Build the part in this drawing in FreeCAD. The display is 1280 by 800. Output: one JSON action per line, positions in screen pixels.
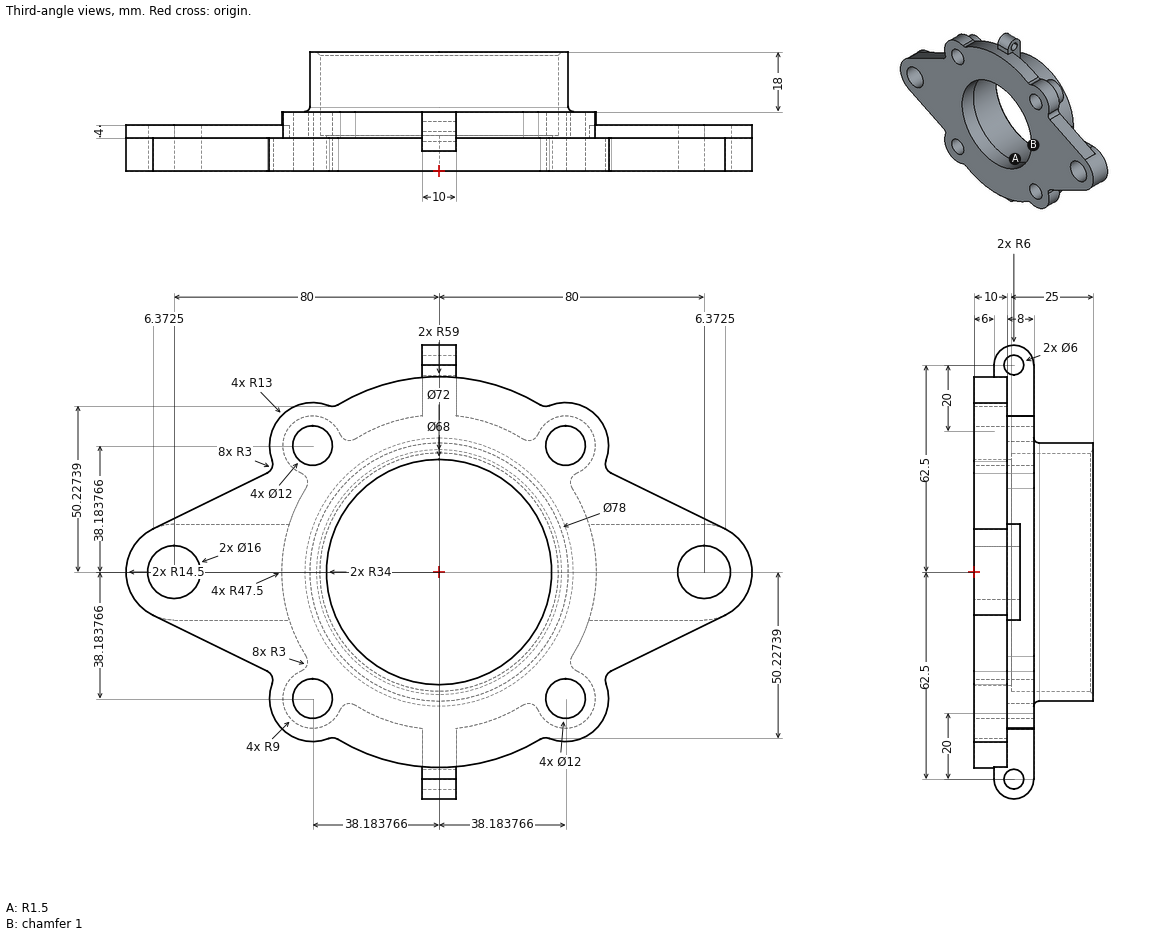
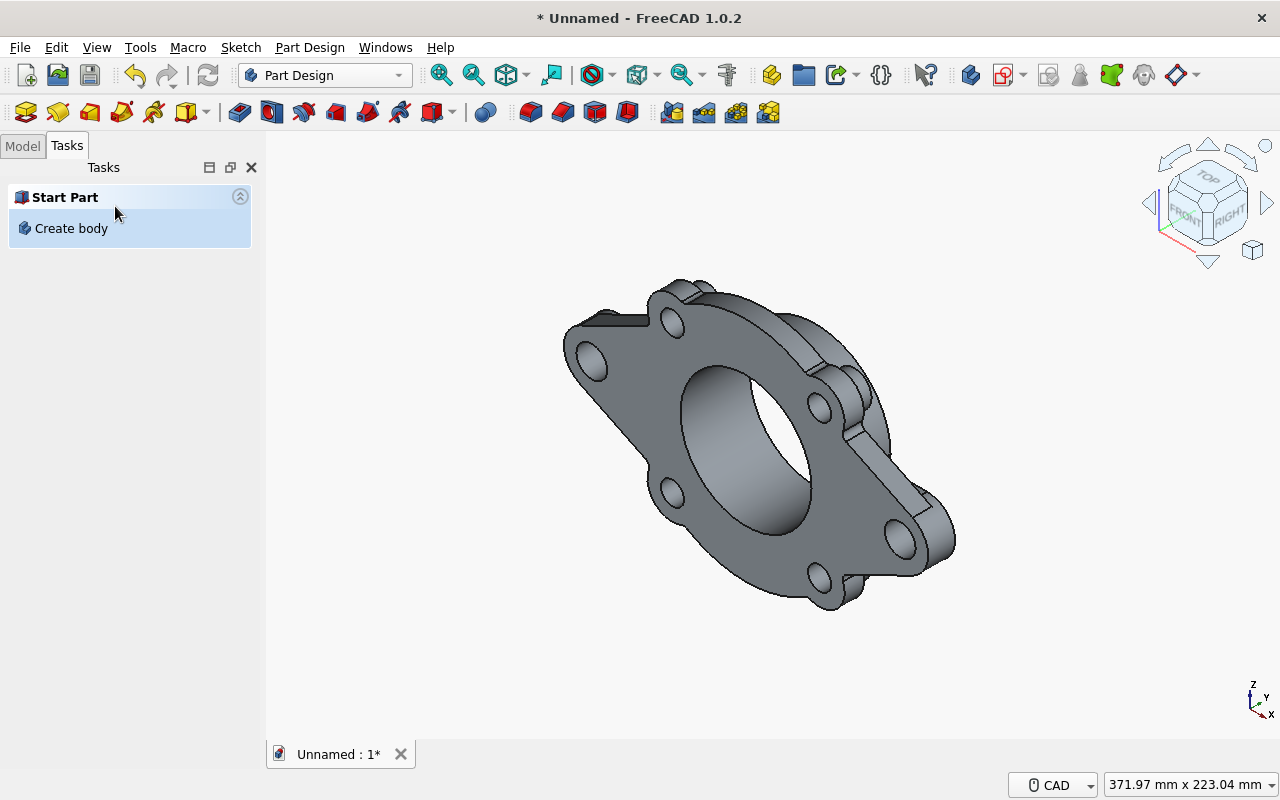
{"action": "key", "text": "2"}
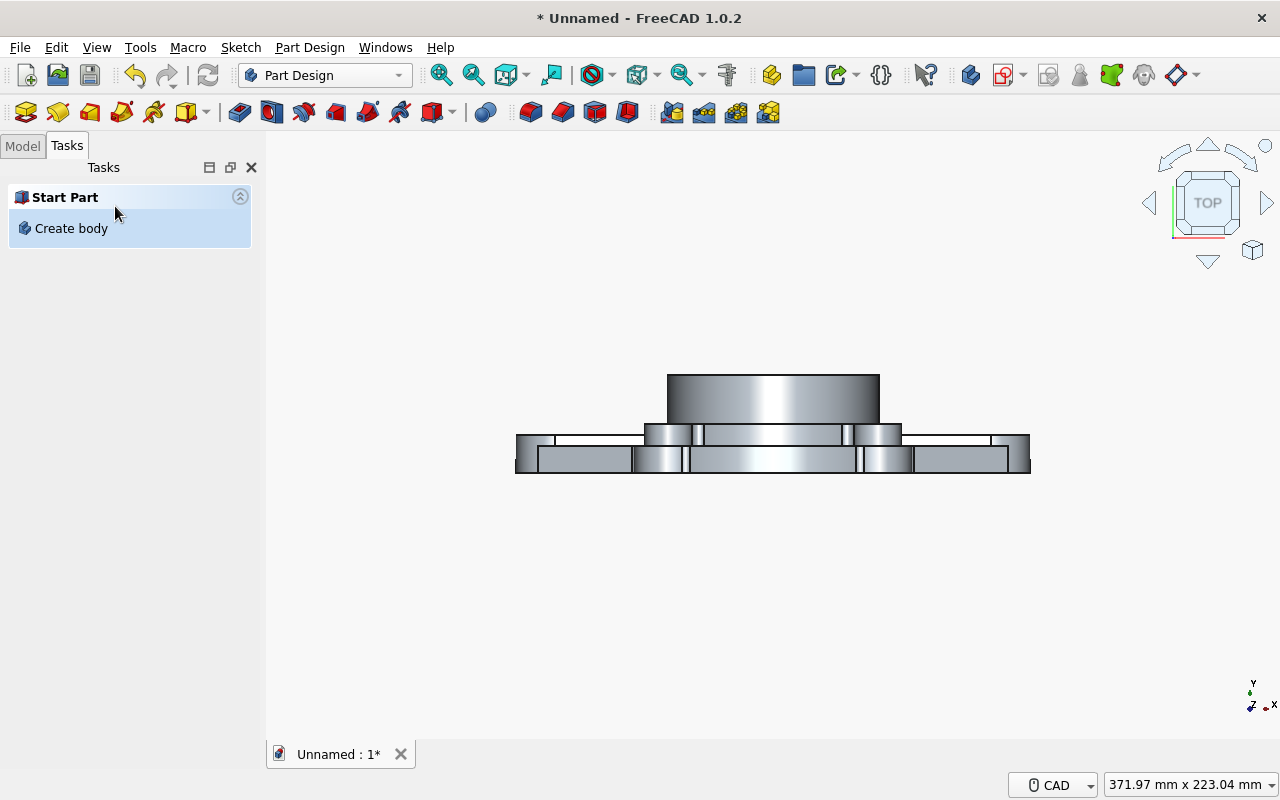
{"action": "key", "text": "1"}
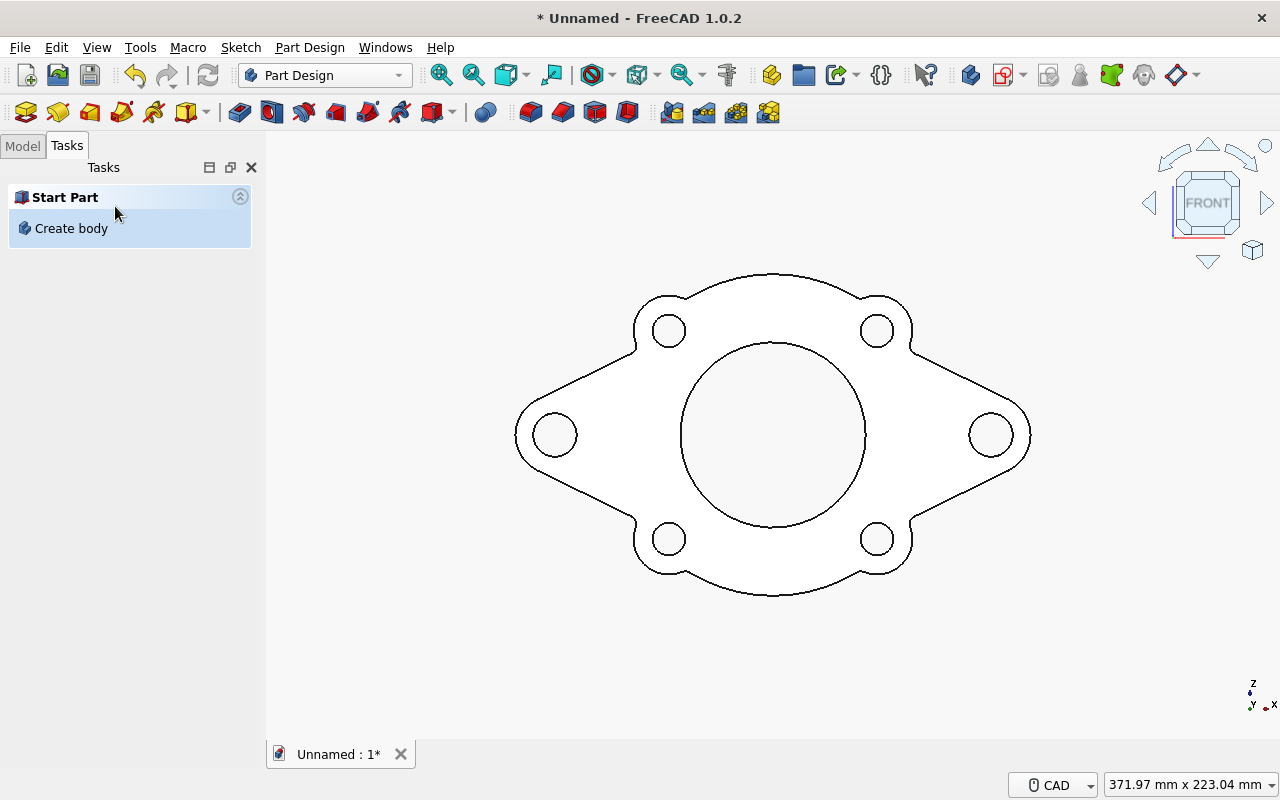
{"action": "key", "text": "3"}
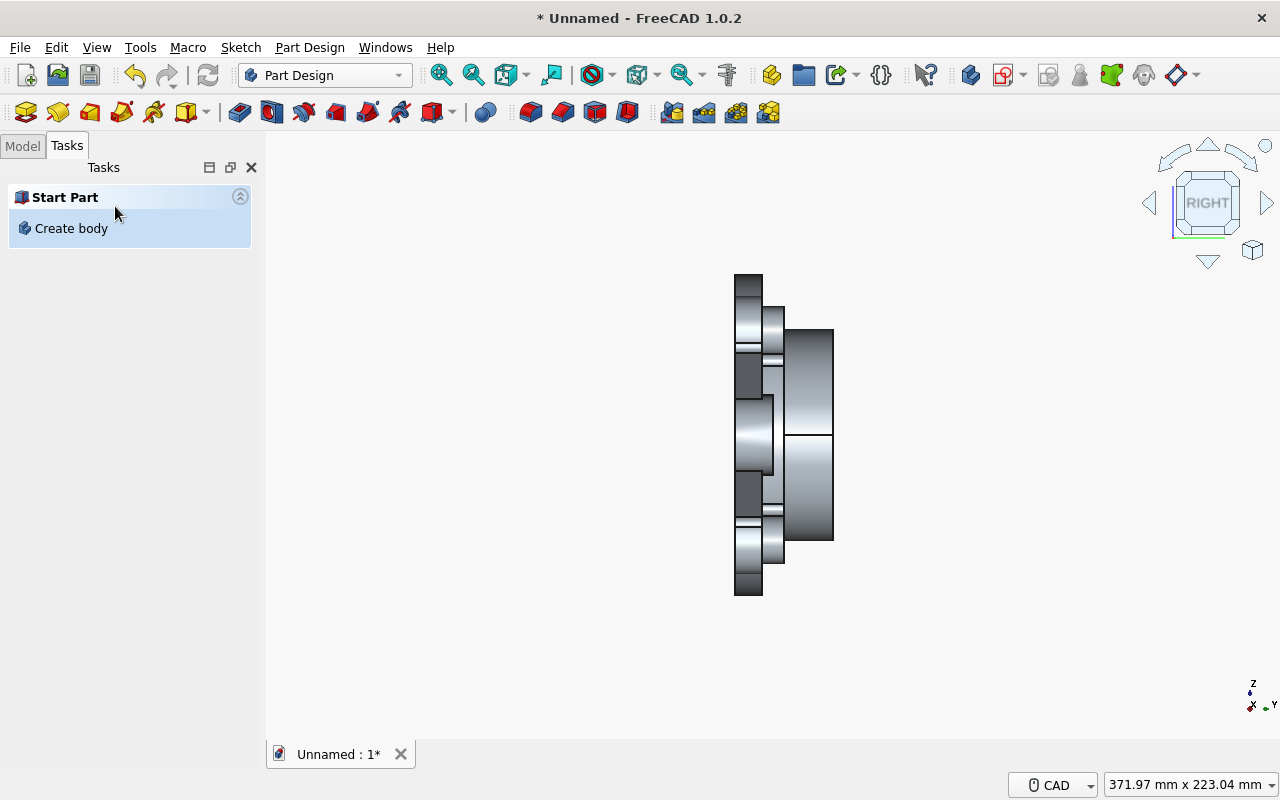
{"action": "key", "text": "5"}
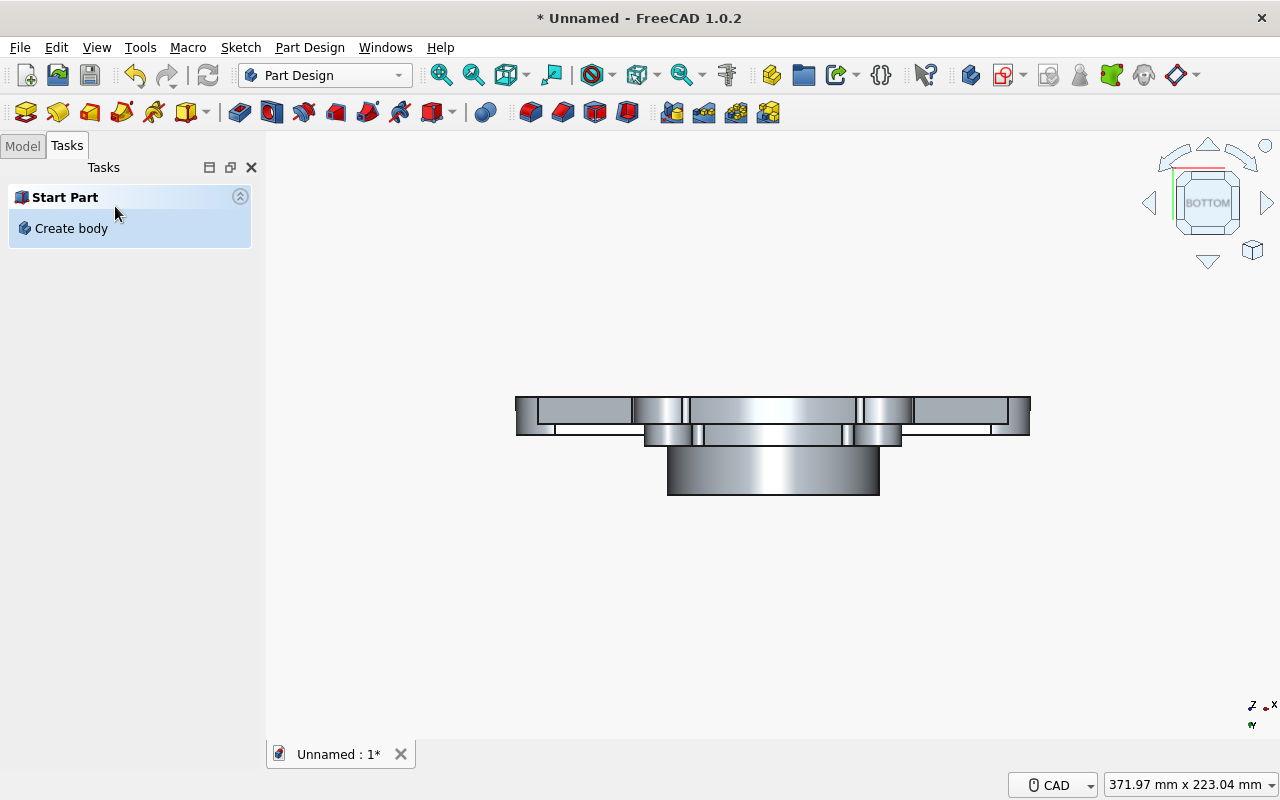
{"action": "key", "text": "4"}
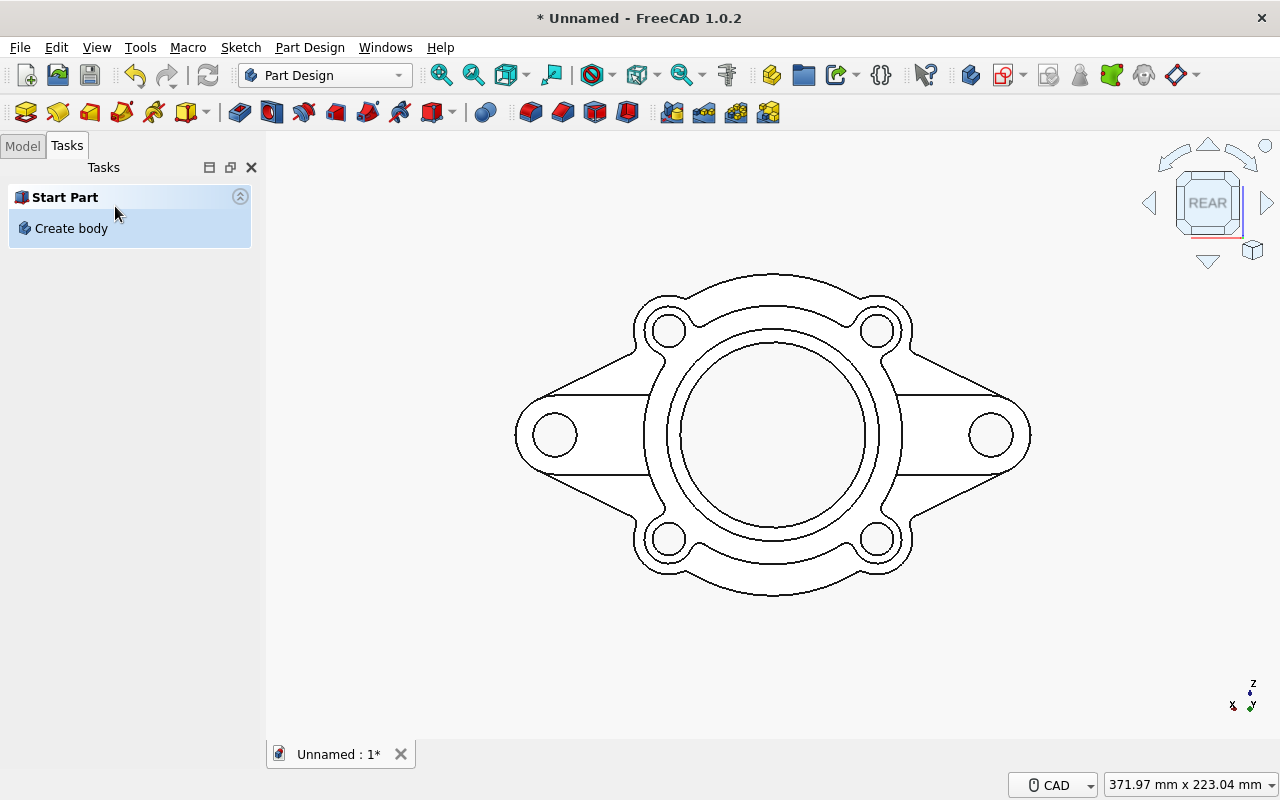
{"action": "key", "text": "6"}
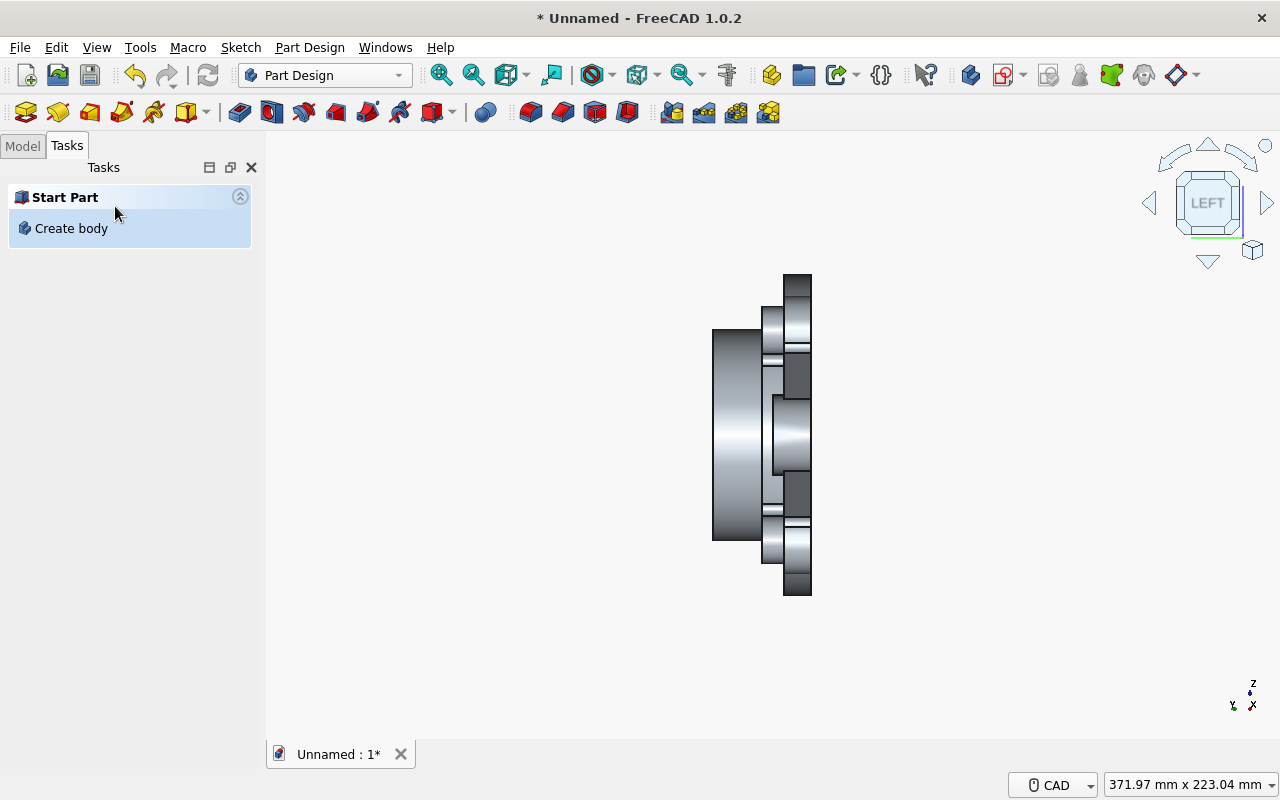
{"action": "key", "text": "v 3"}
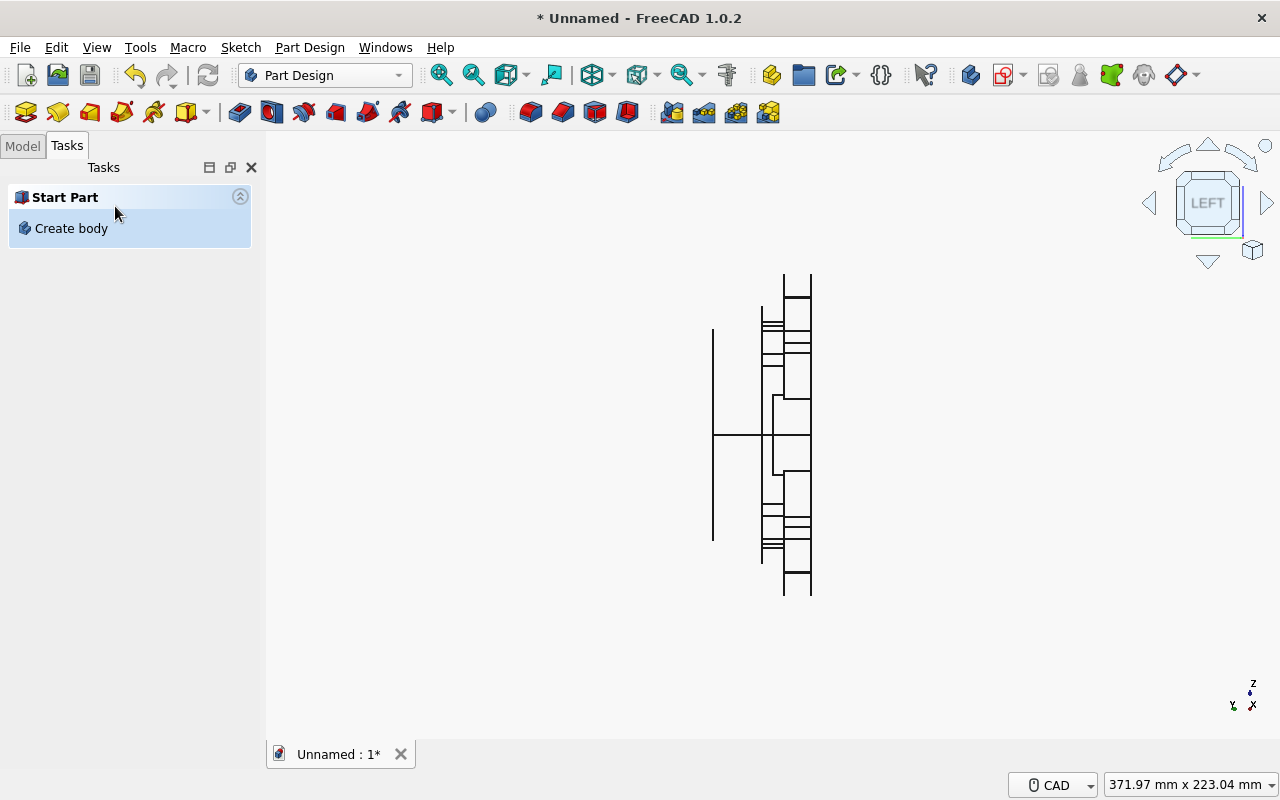
{"action": "key", "text": "0"}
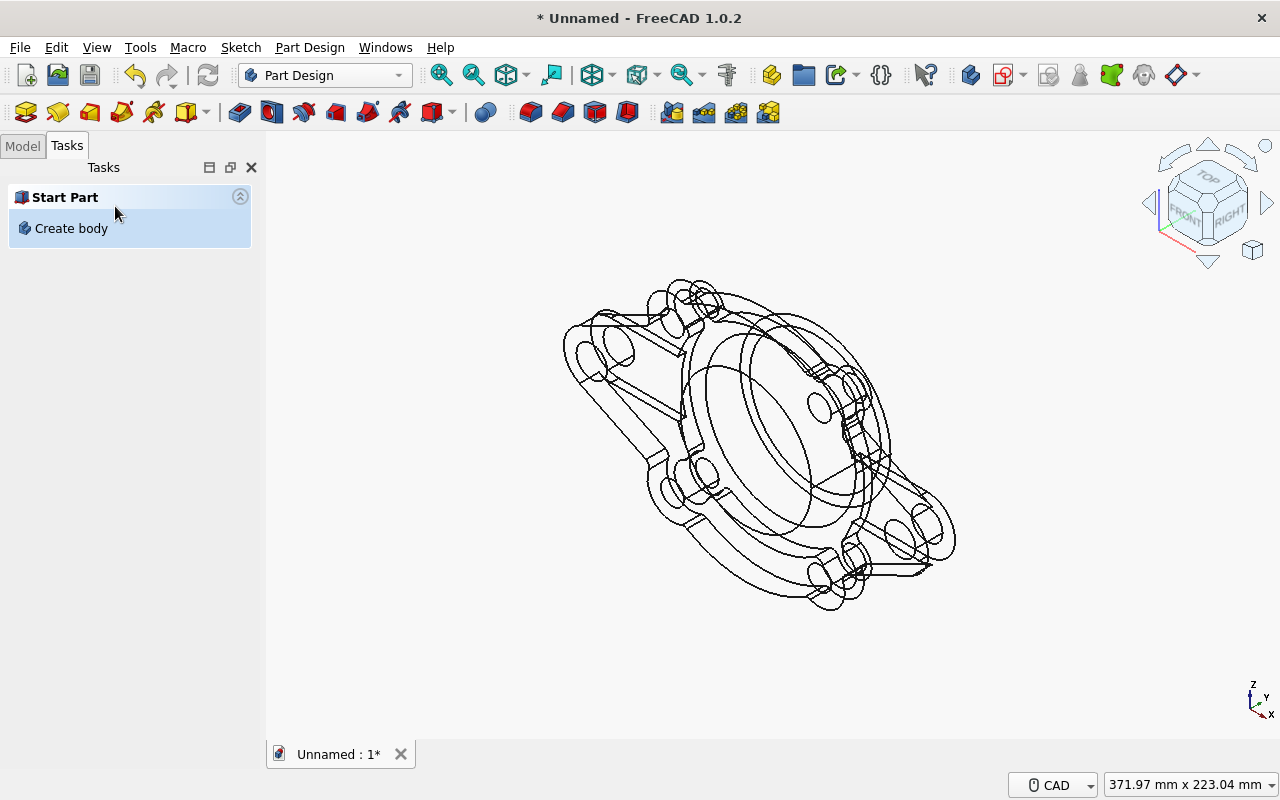
{"action": "left_click", "coordinate": [706, 386]}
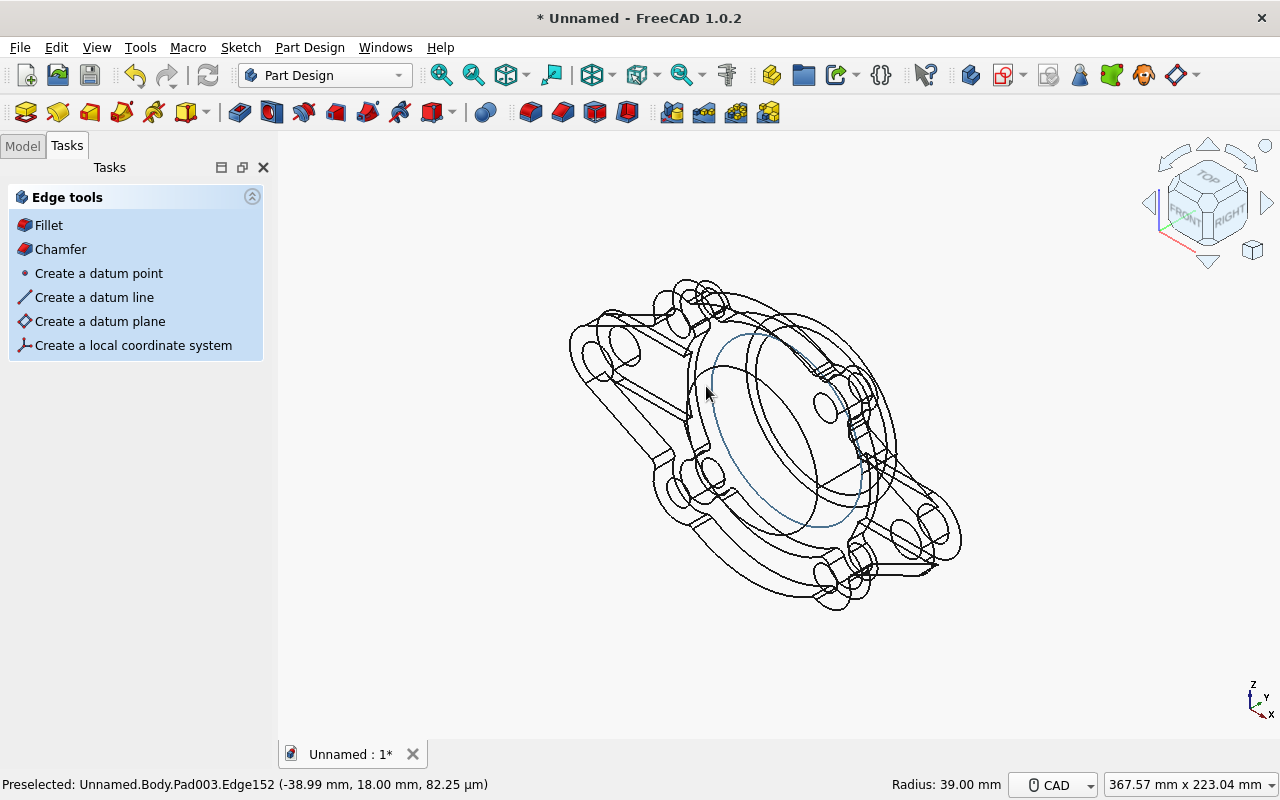
{"action": "key", "text": "v 1"}